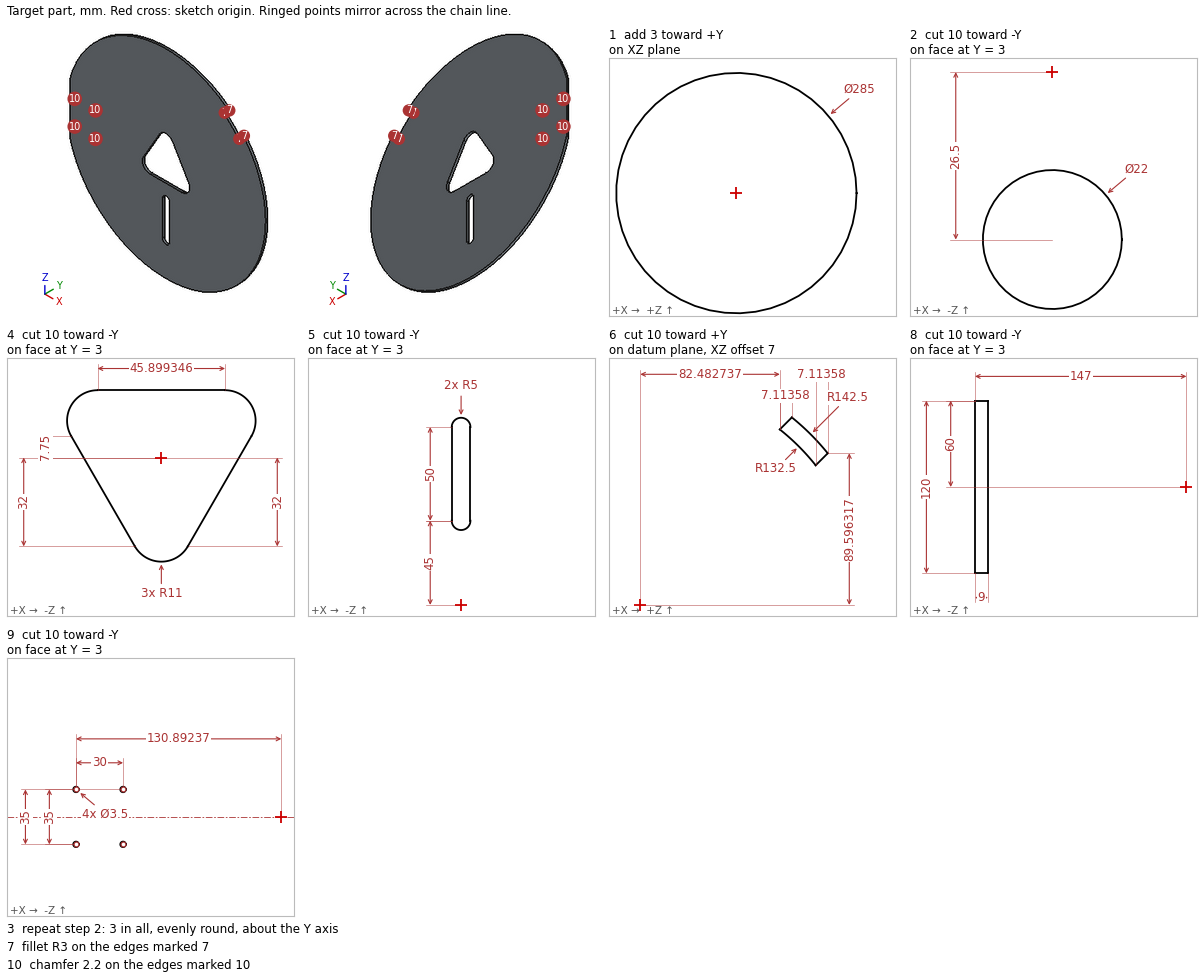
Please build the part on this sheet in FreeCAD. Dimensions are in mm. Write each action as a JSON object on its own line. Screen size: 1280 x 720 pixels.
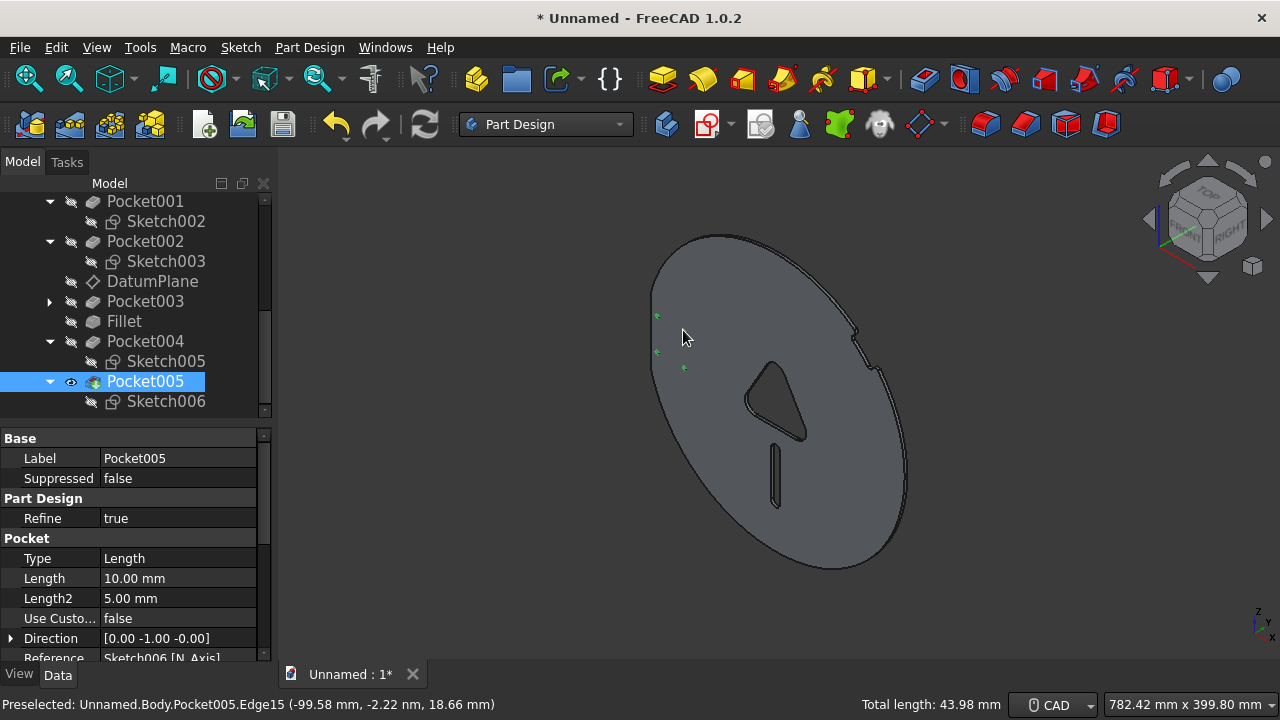
{"action": "left_click", "coordinate": [1026, 124]}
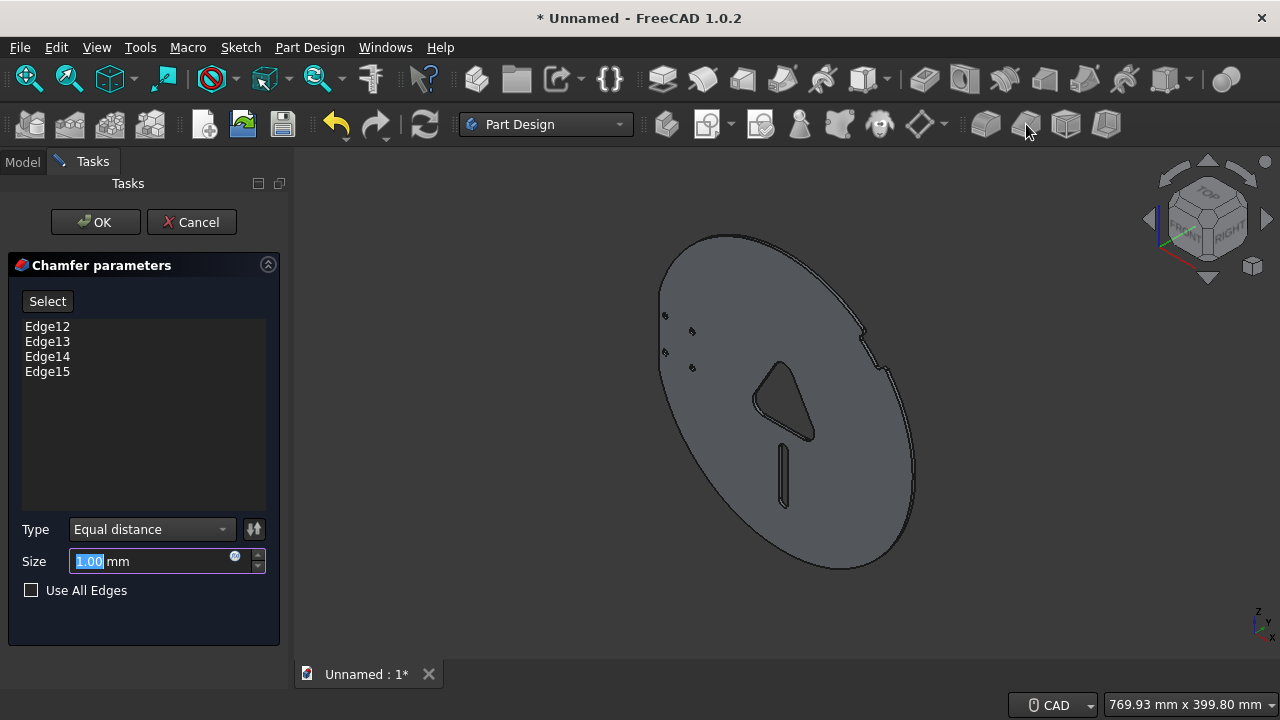
{"action": "type", "text": "2.2"}
{"action": "key", "text": "Tab"}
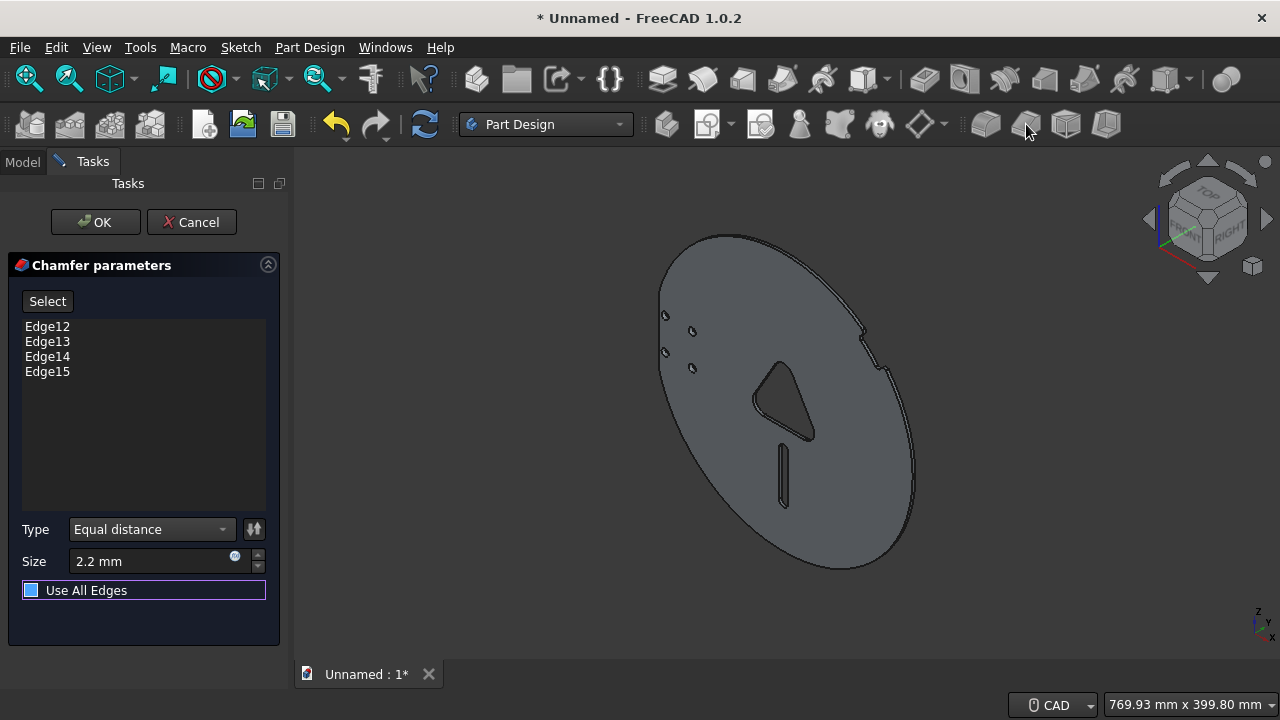
{"action": "left_click", "coordinate": [96, 222]}